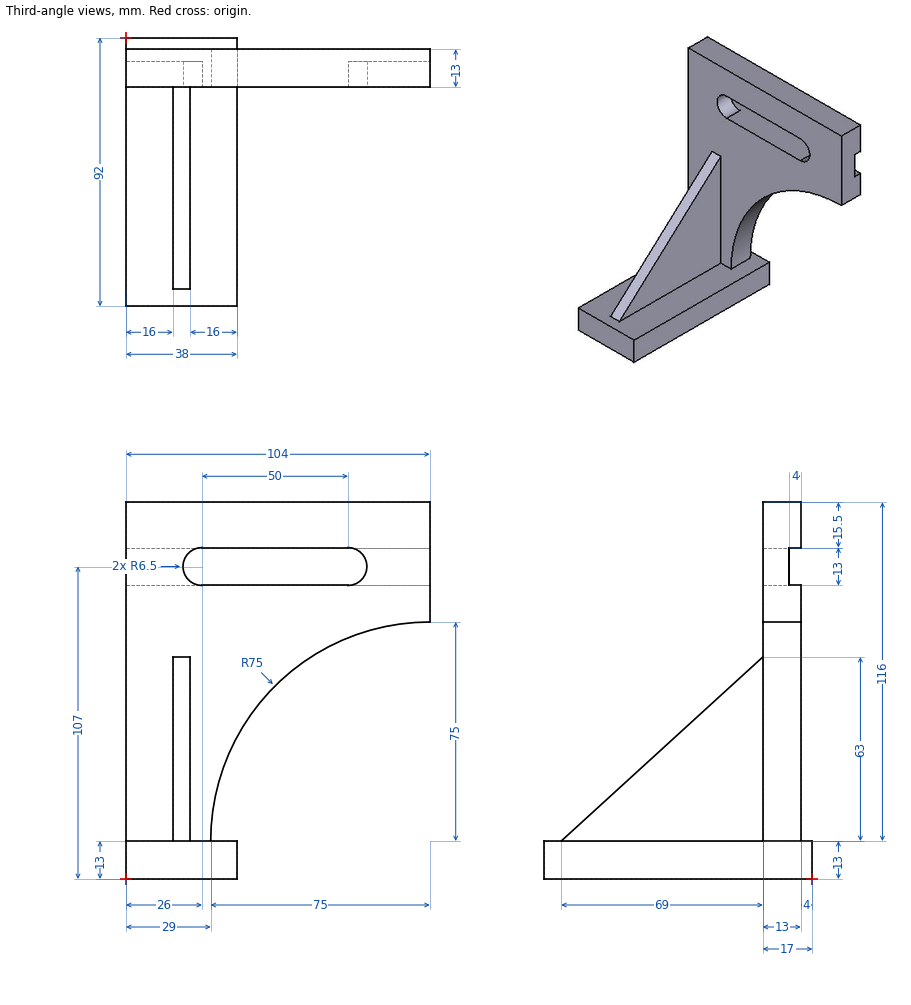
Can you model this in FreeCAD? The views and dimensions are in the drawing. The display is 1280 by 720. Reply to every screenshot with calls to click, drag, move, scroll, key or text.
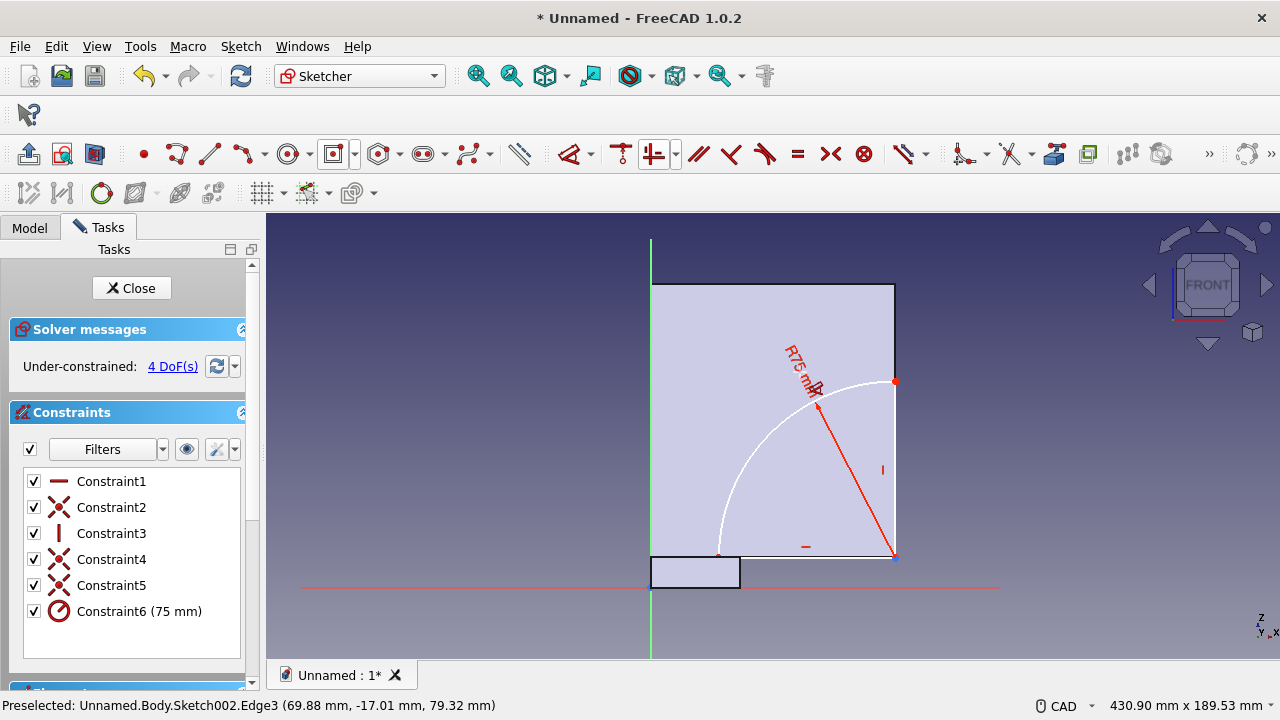
click(772, 558)
click(807, 524)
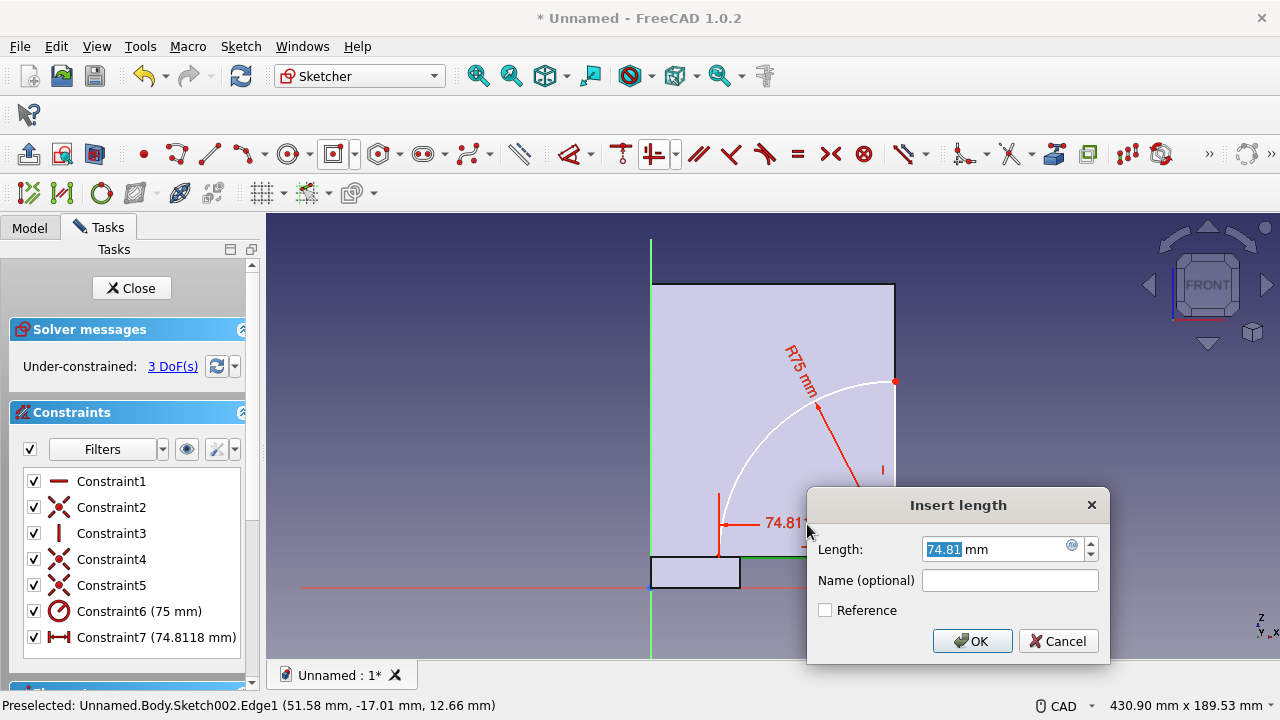
text(75)
key(Return)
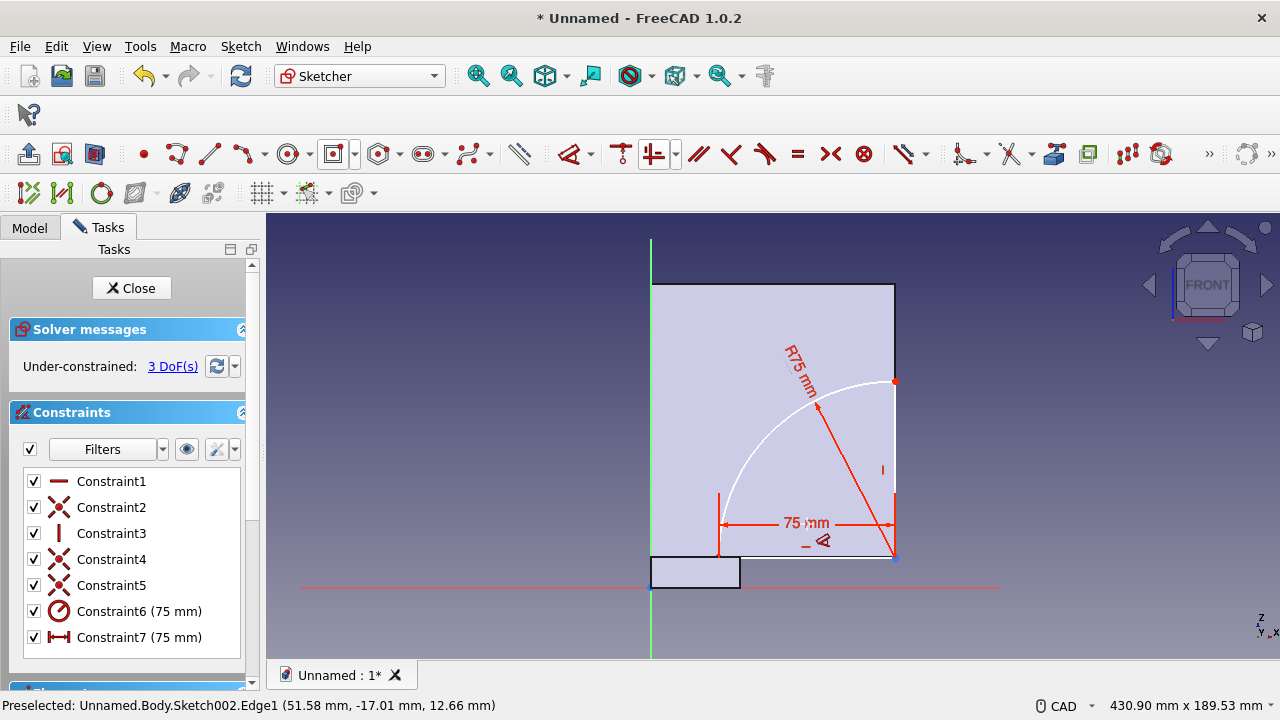
click(895, 505)
click(929, 470)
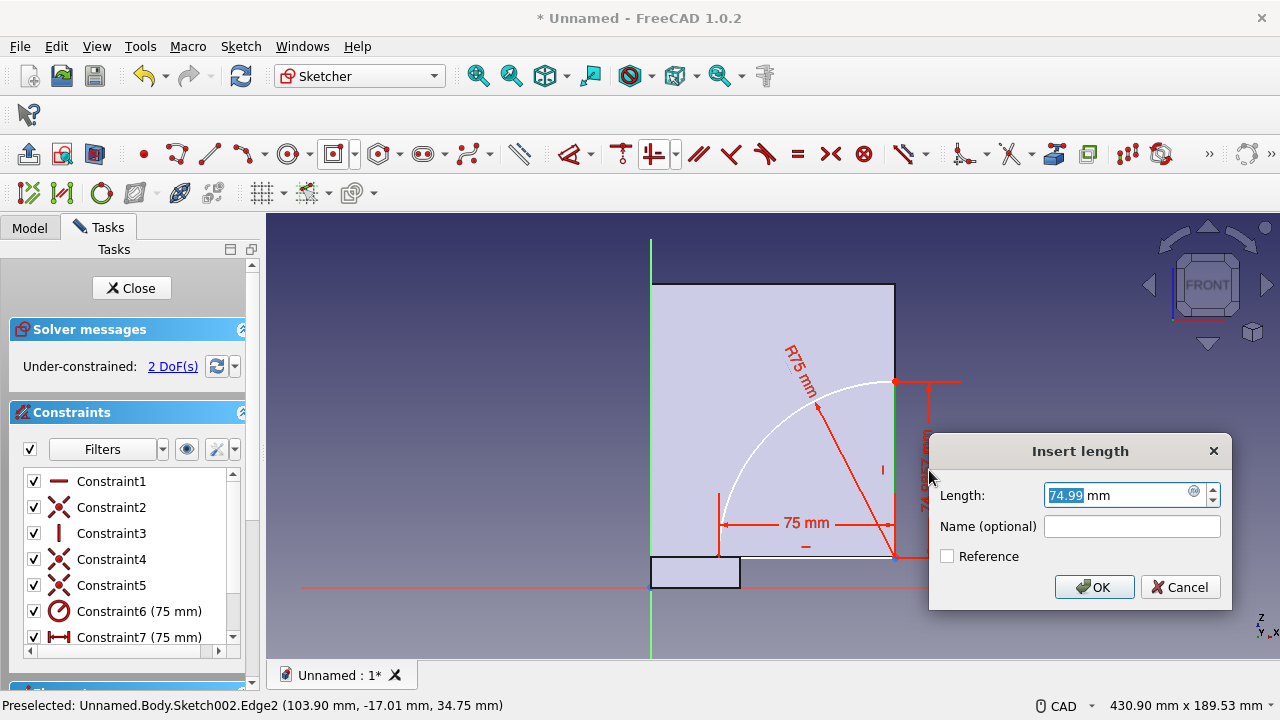
text(75)
key(Return)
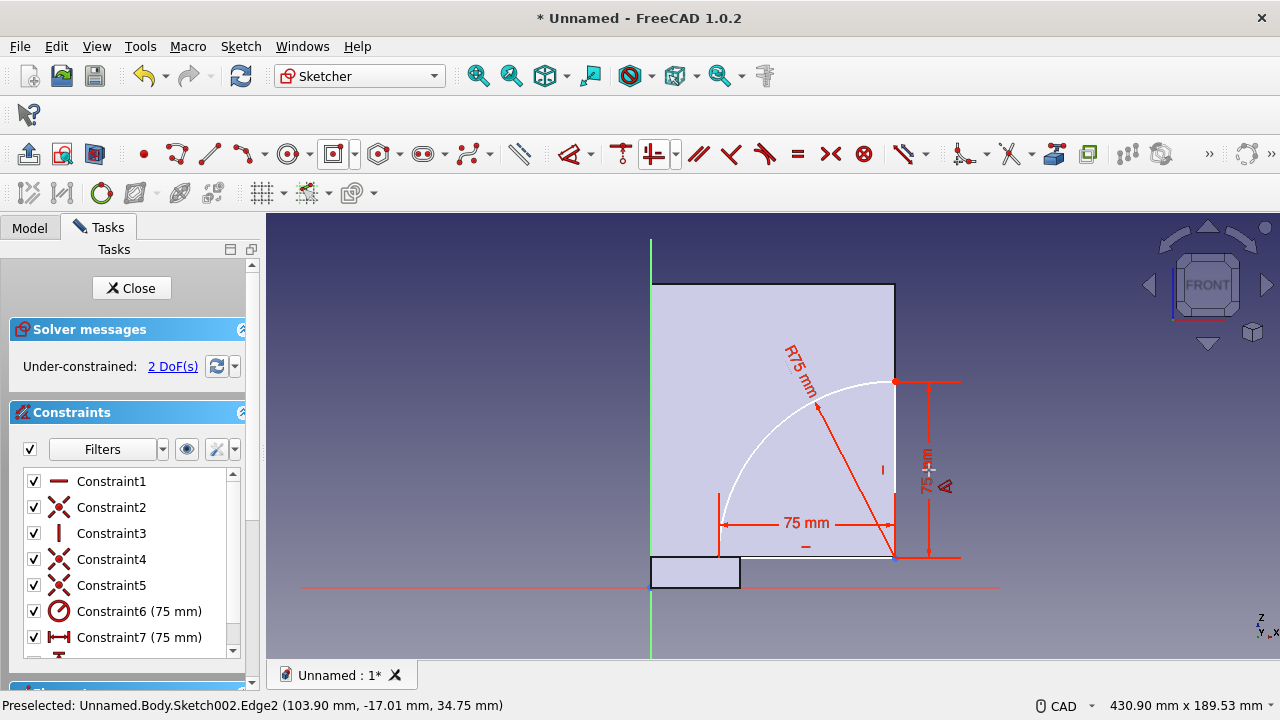
click(719, 558)
click(685, 622)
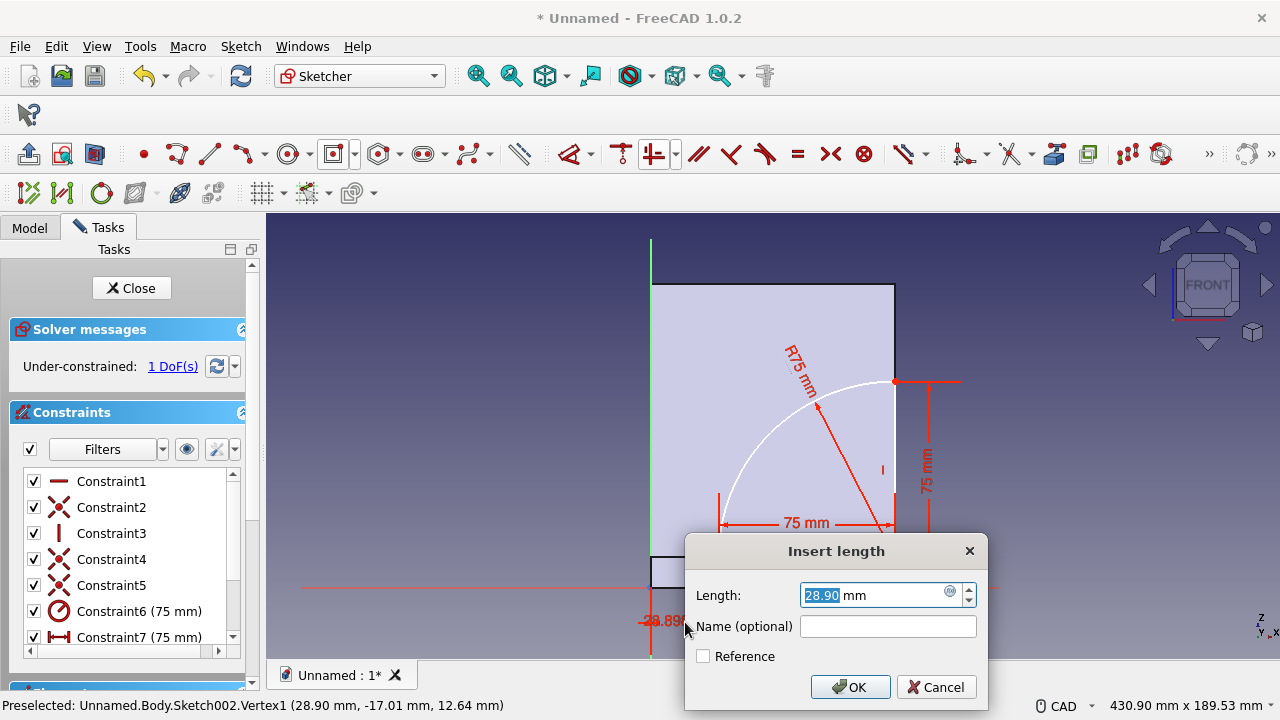
text(29)
key(Return)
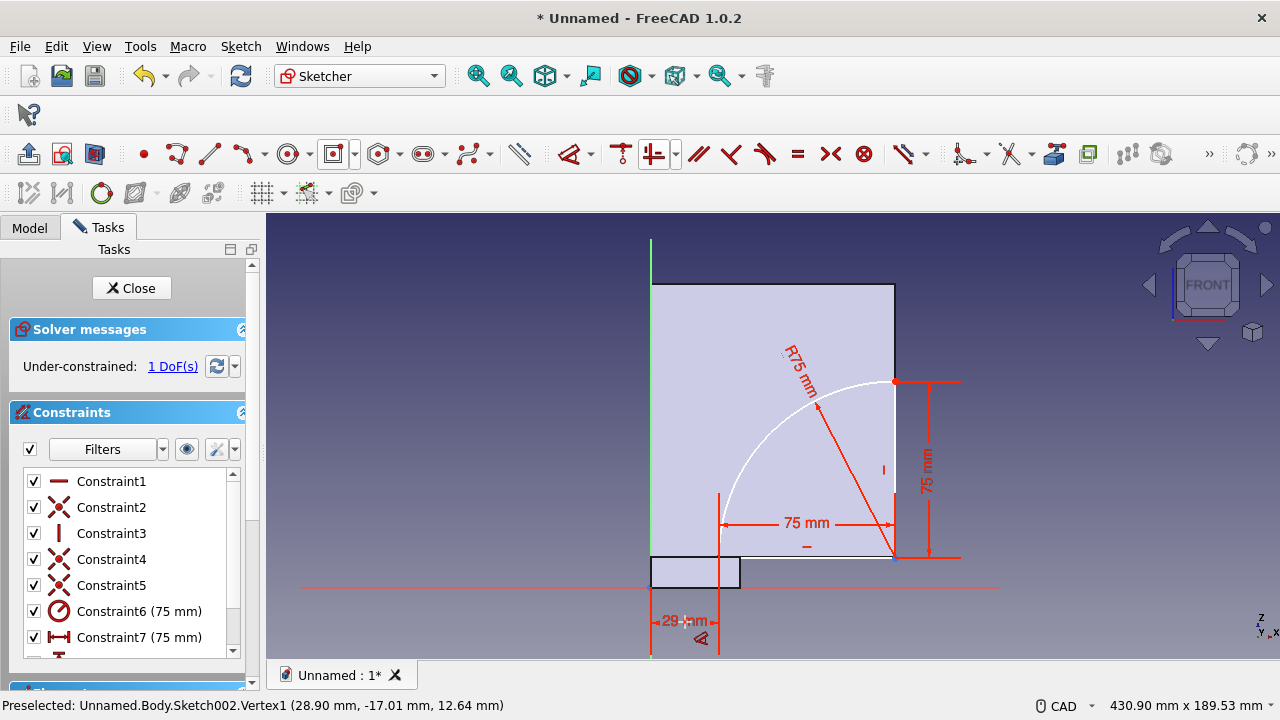
scroll(719, 558, up, 2)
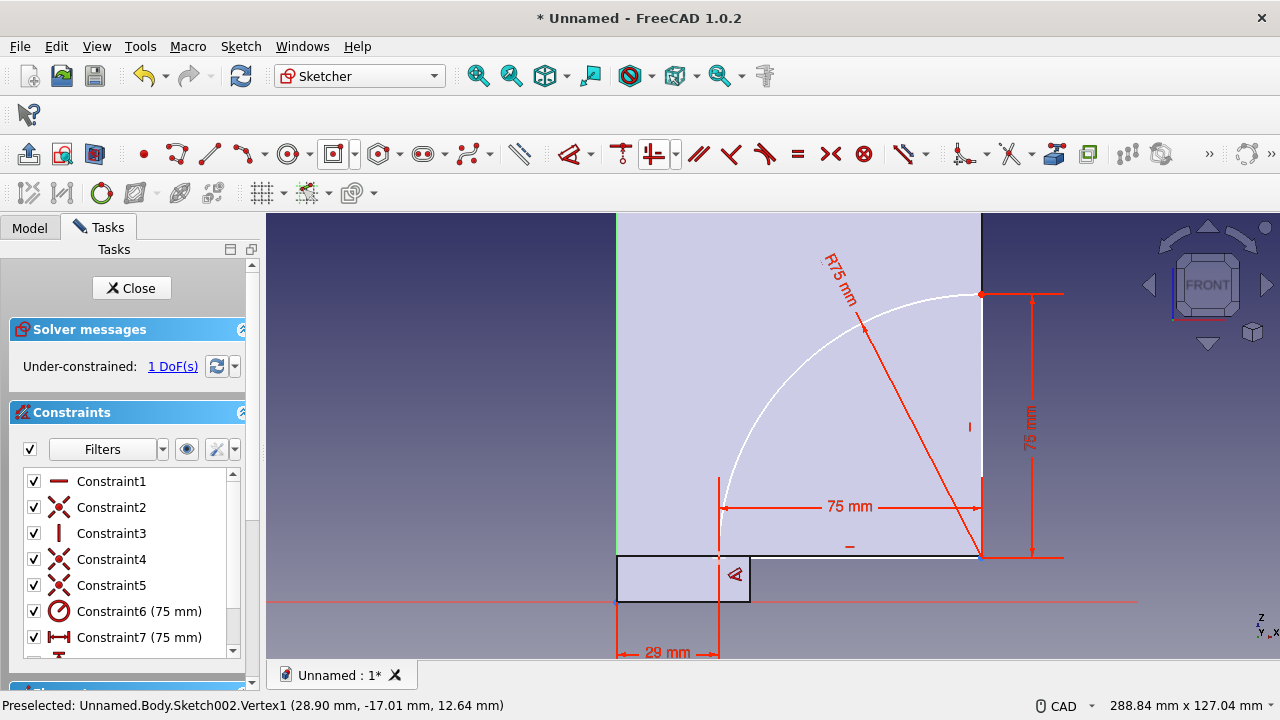
click(719, 558)
click(583, 580)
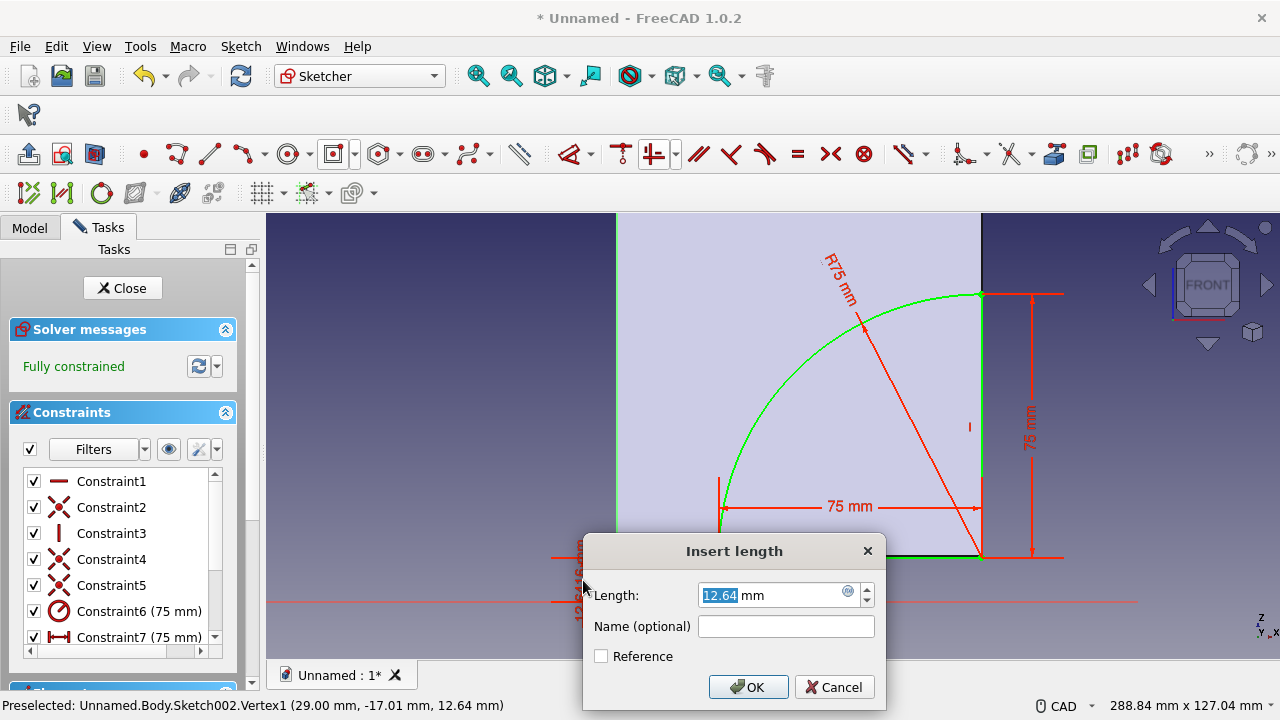
text(13)
key(Return)
key(Escape)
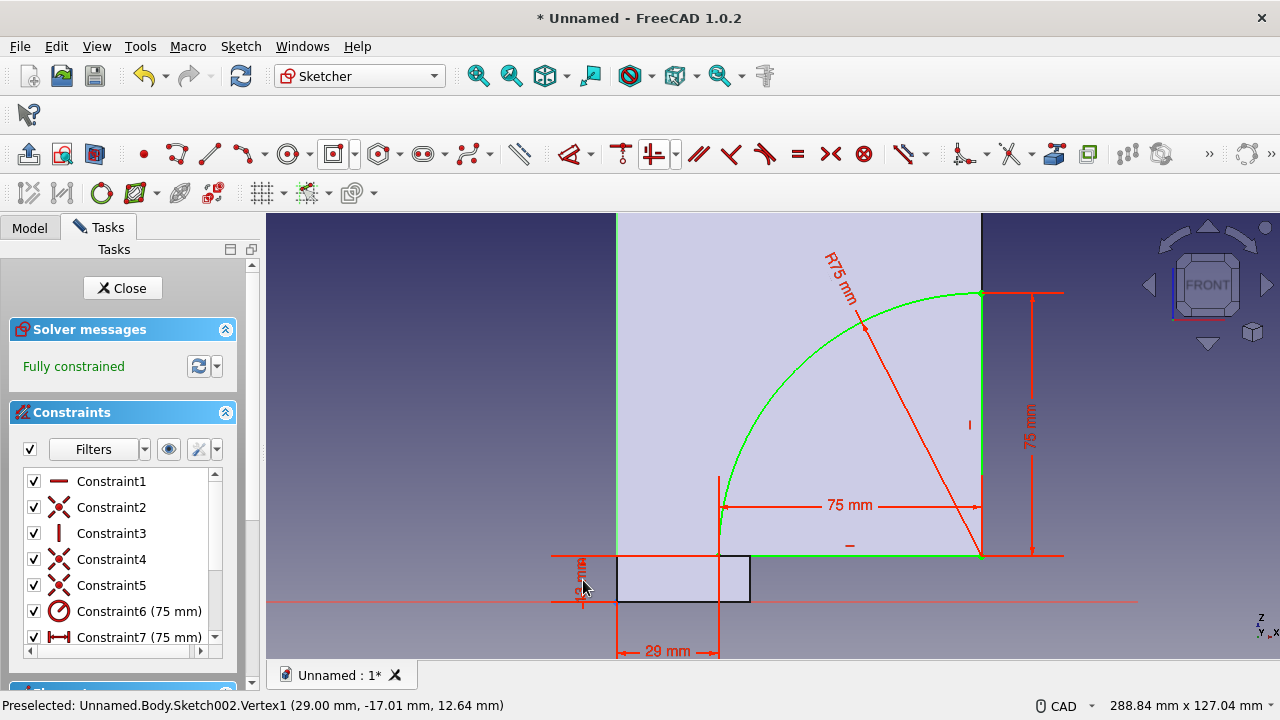
click(123, 288)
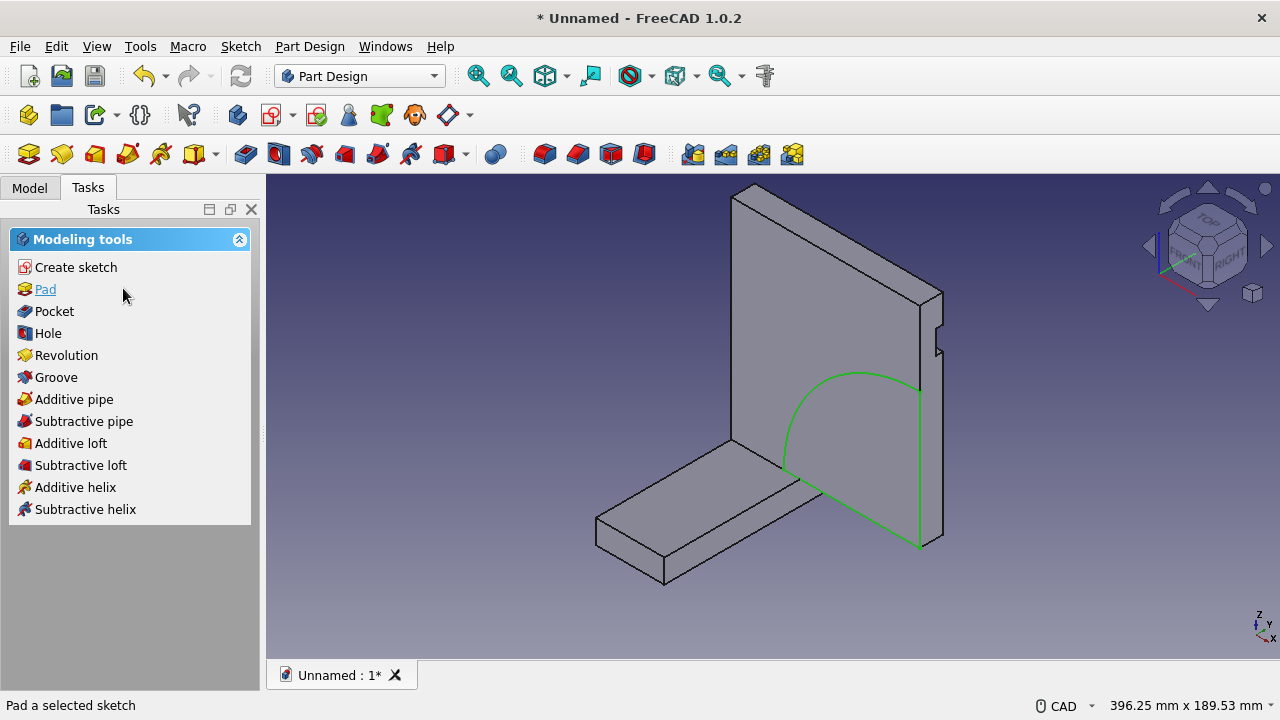
click(246, 154)